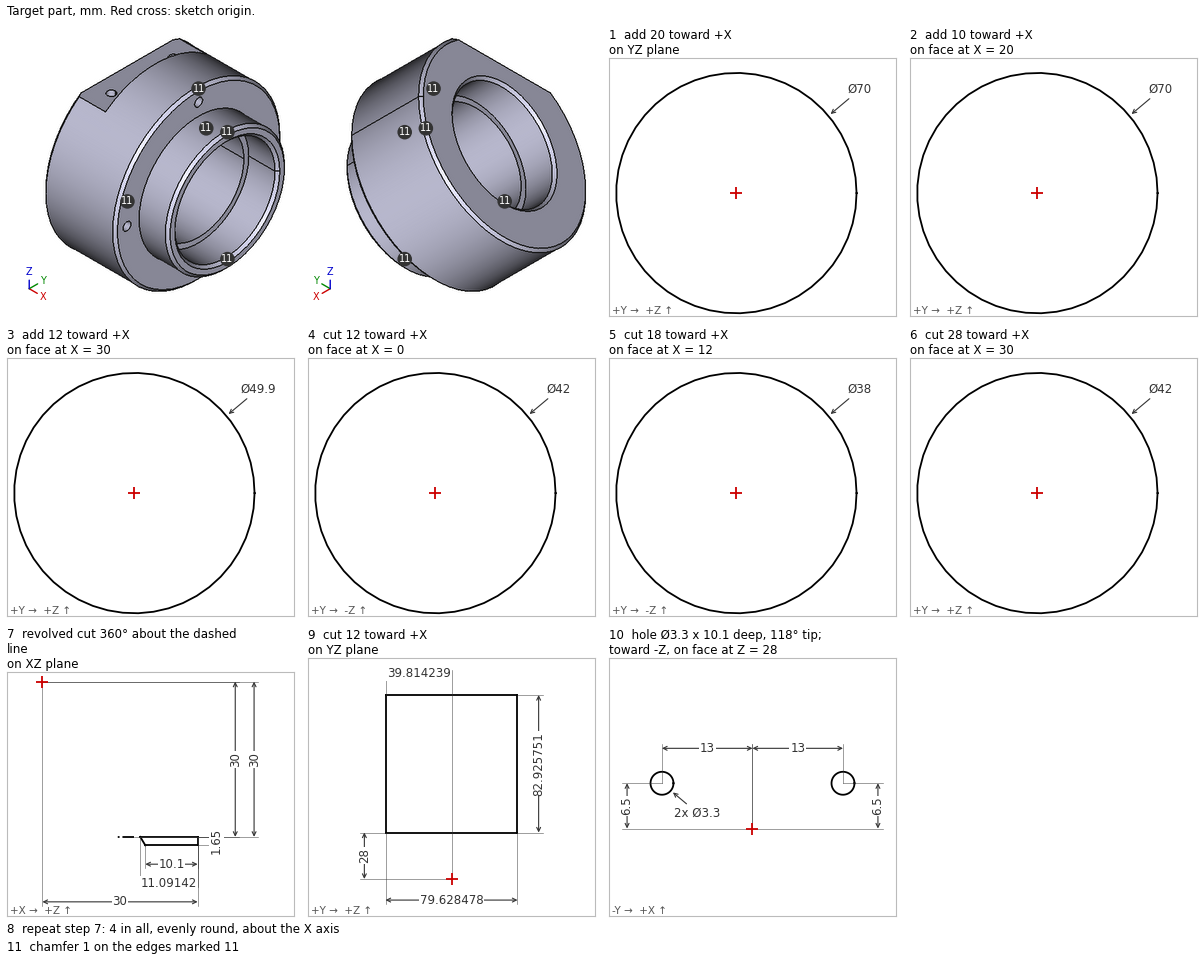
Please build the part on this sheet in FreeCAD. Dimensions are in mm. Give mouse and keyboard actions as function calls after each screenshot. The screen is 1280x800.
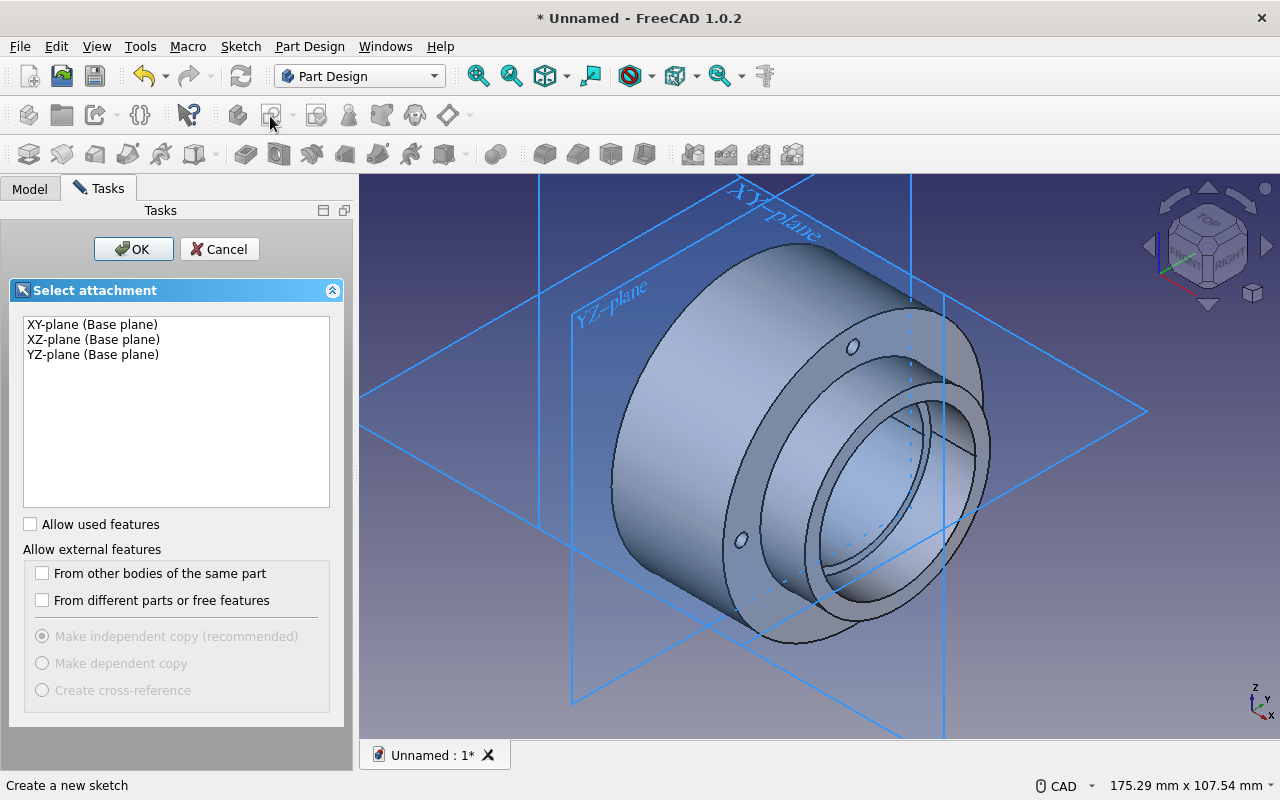
click(84, 354)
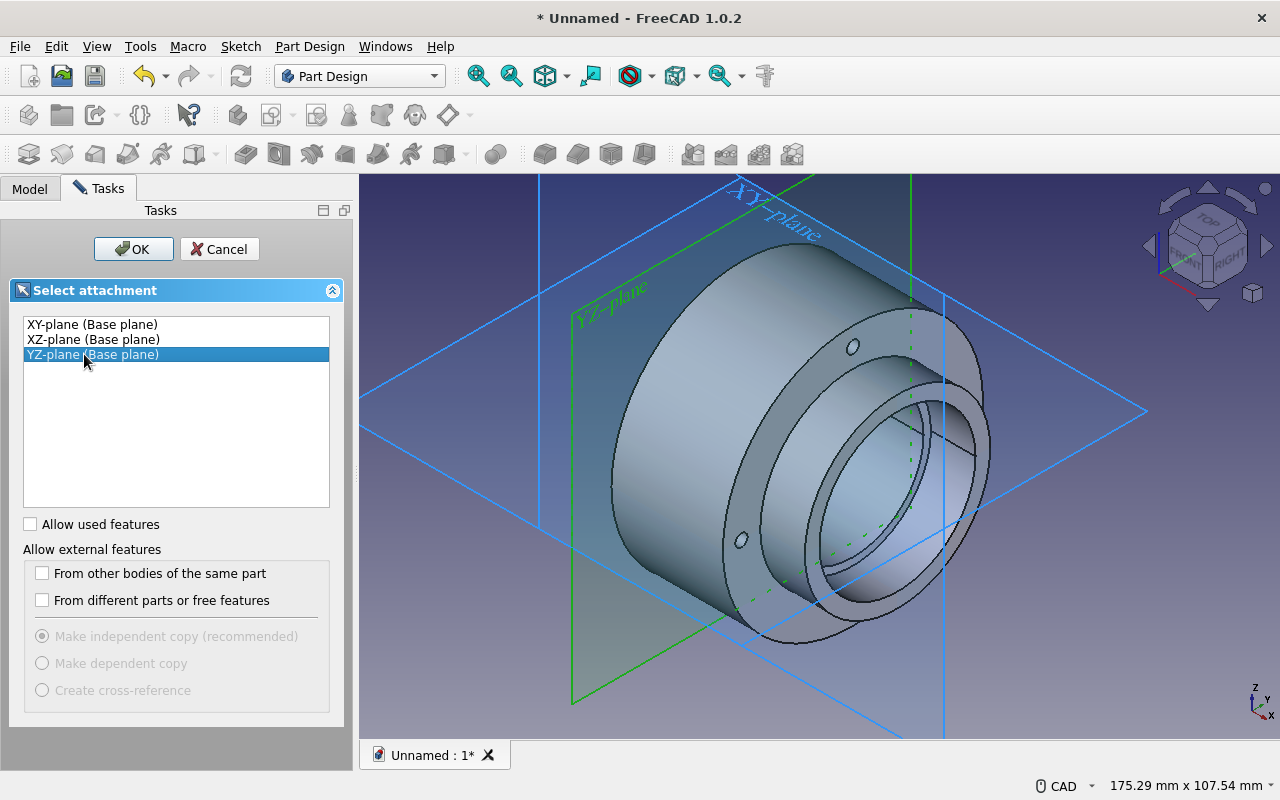
click(134, 249)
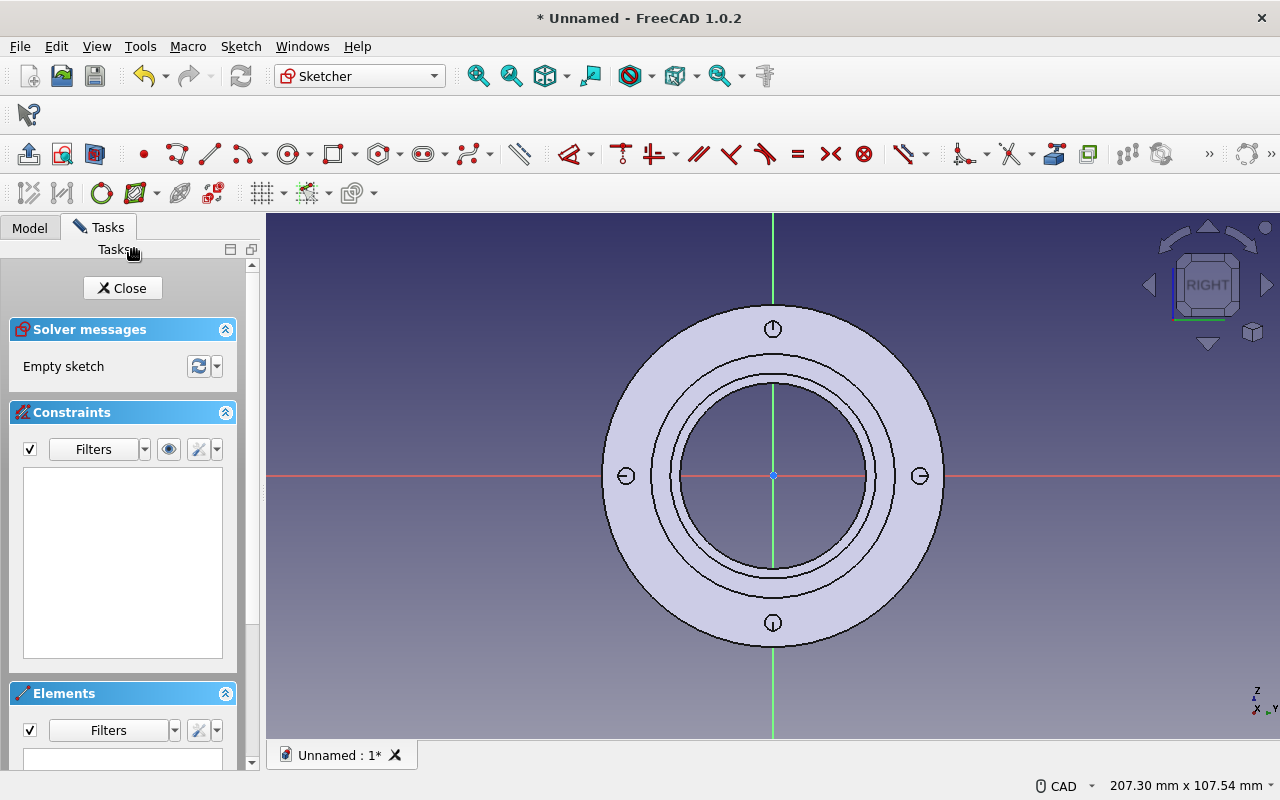
click(95, 154)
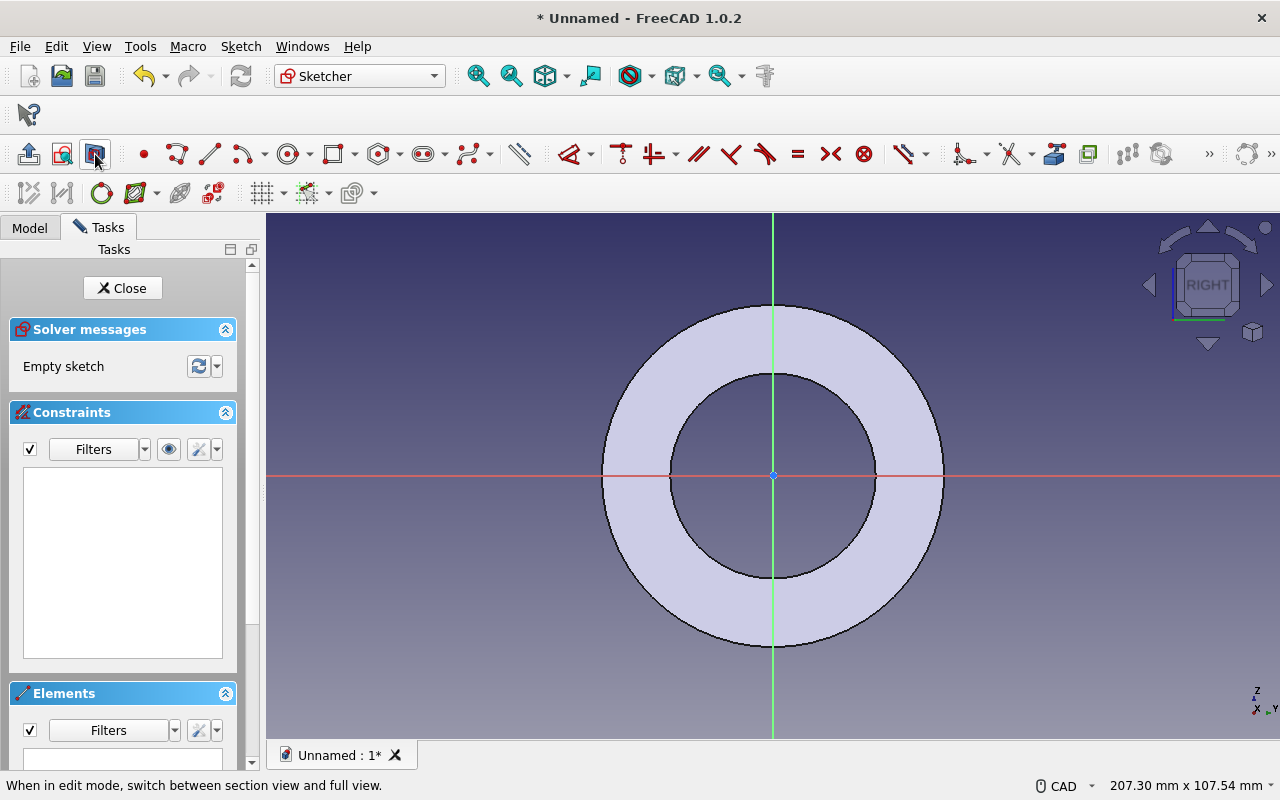
scroll(621, 711, down, 3)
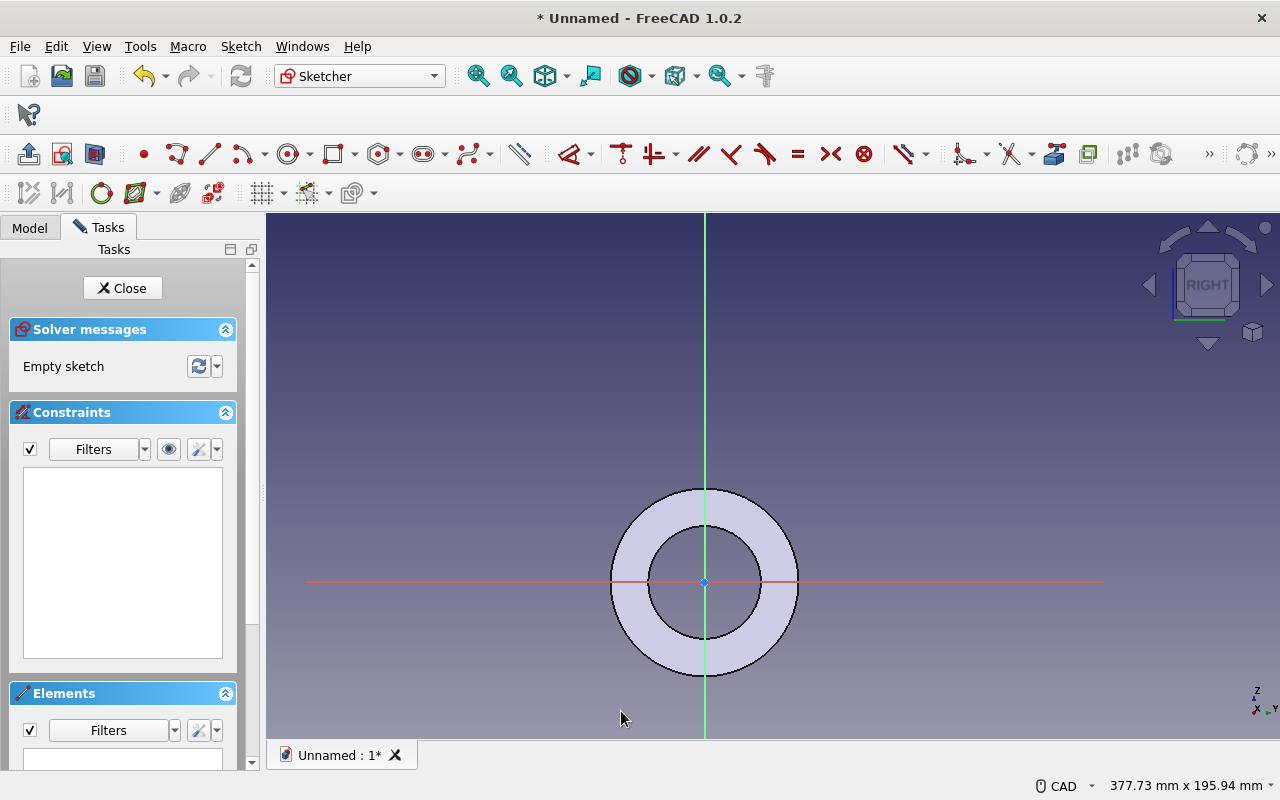
click(332, 154)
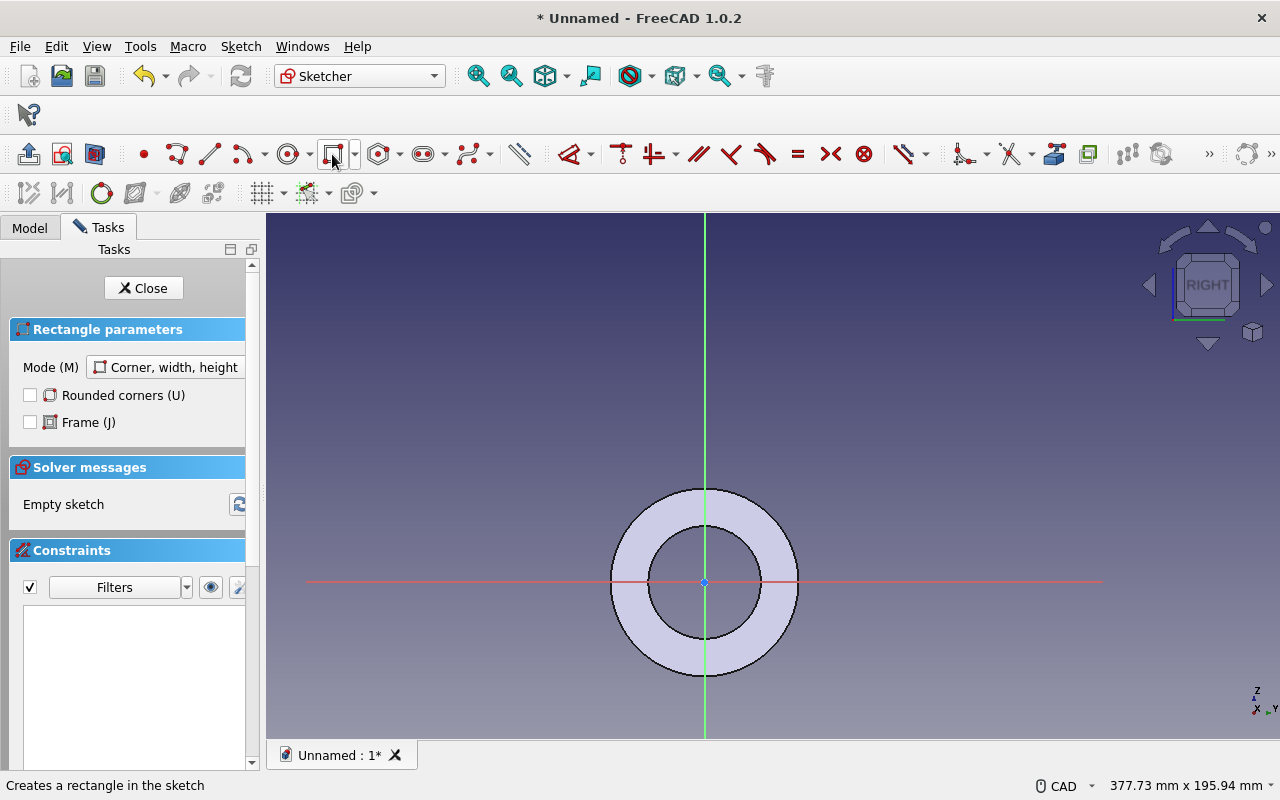
click(598, 285)
move(811, 507)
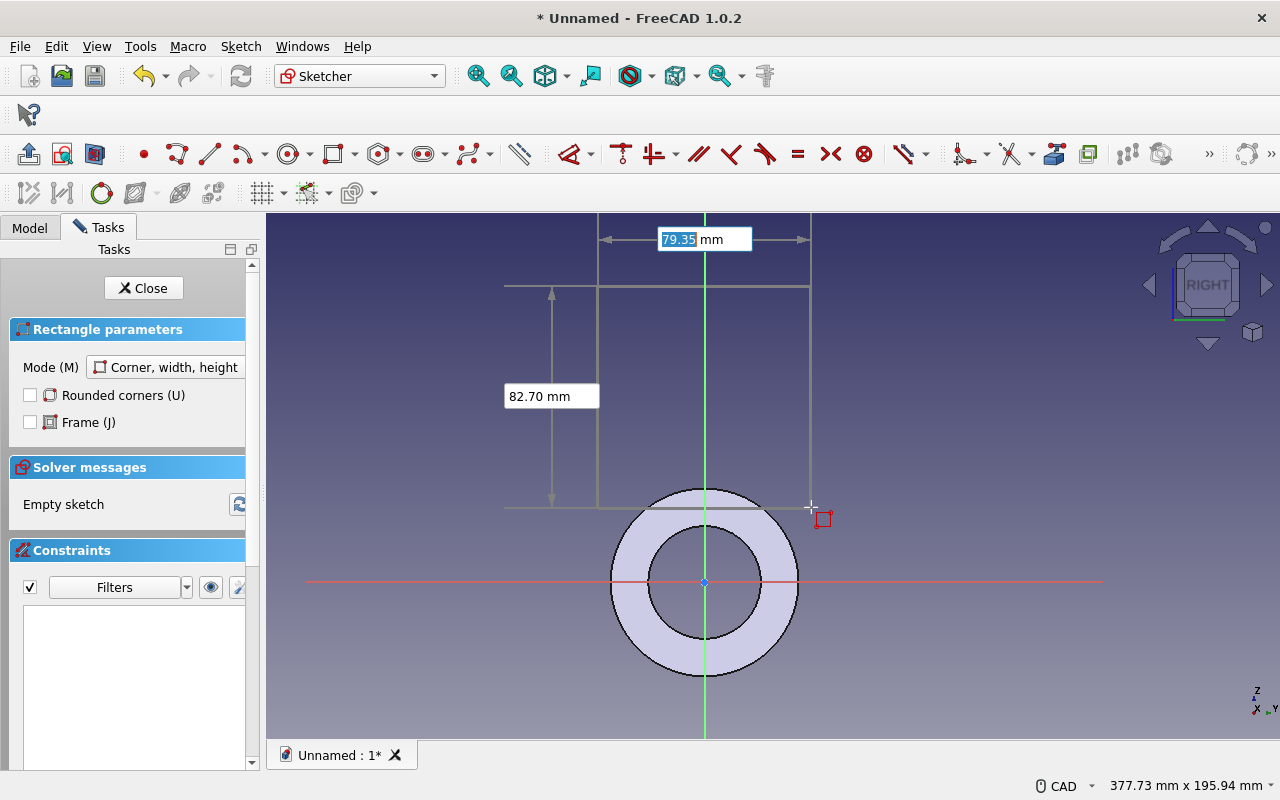
text(79.628478)
key(Tab)
text(82.925751)
key(Return)
key(Escape)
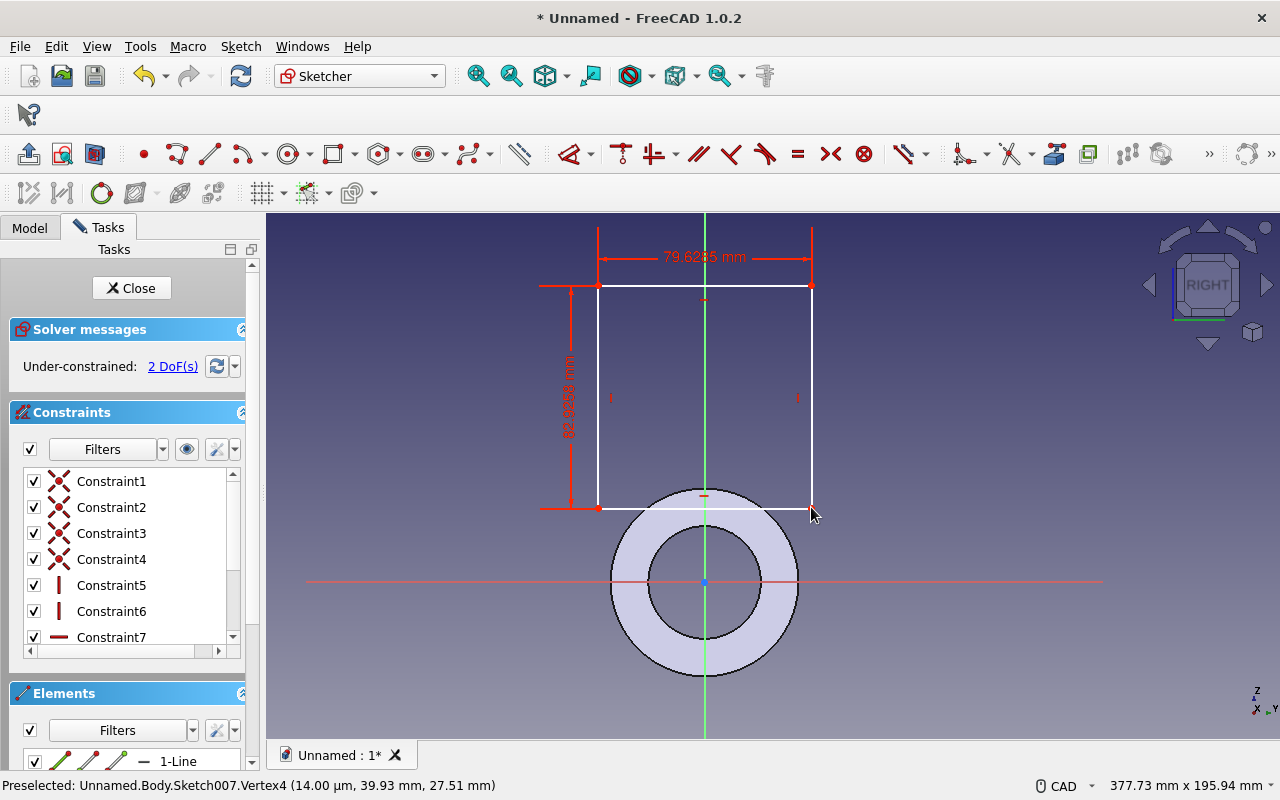
click(568, 154)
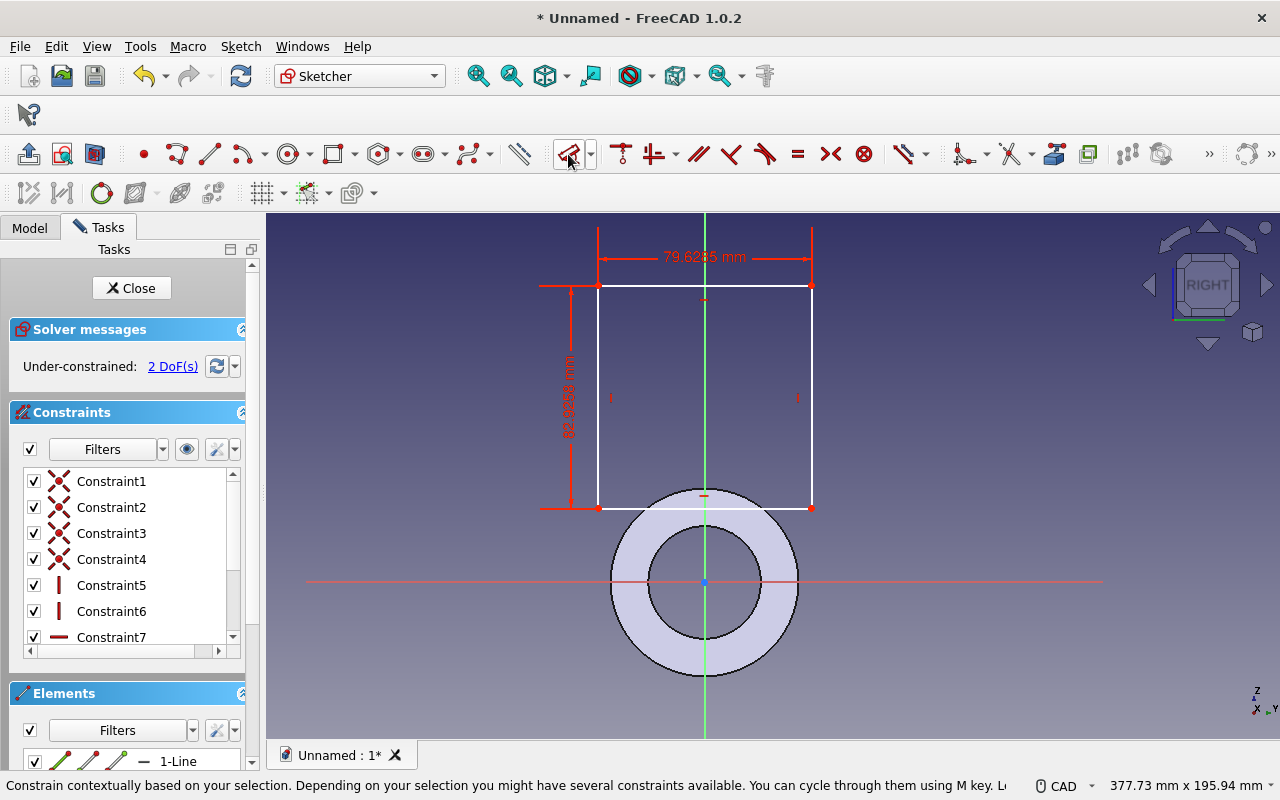
click(598, 509)
click(564, 546)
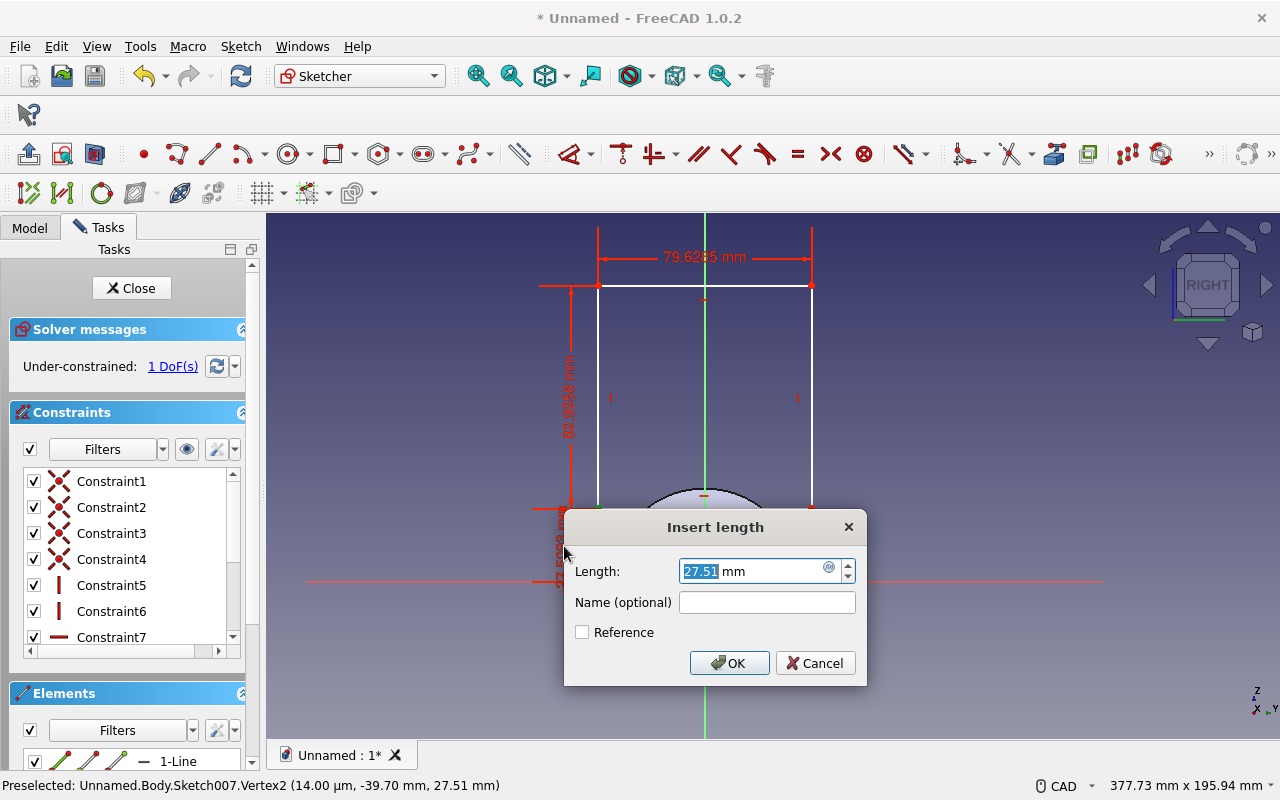
text(28)
key(Return)